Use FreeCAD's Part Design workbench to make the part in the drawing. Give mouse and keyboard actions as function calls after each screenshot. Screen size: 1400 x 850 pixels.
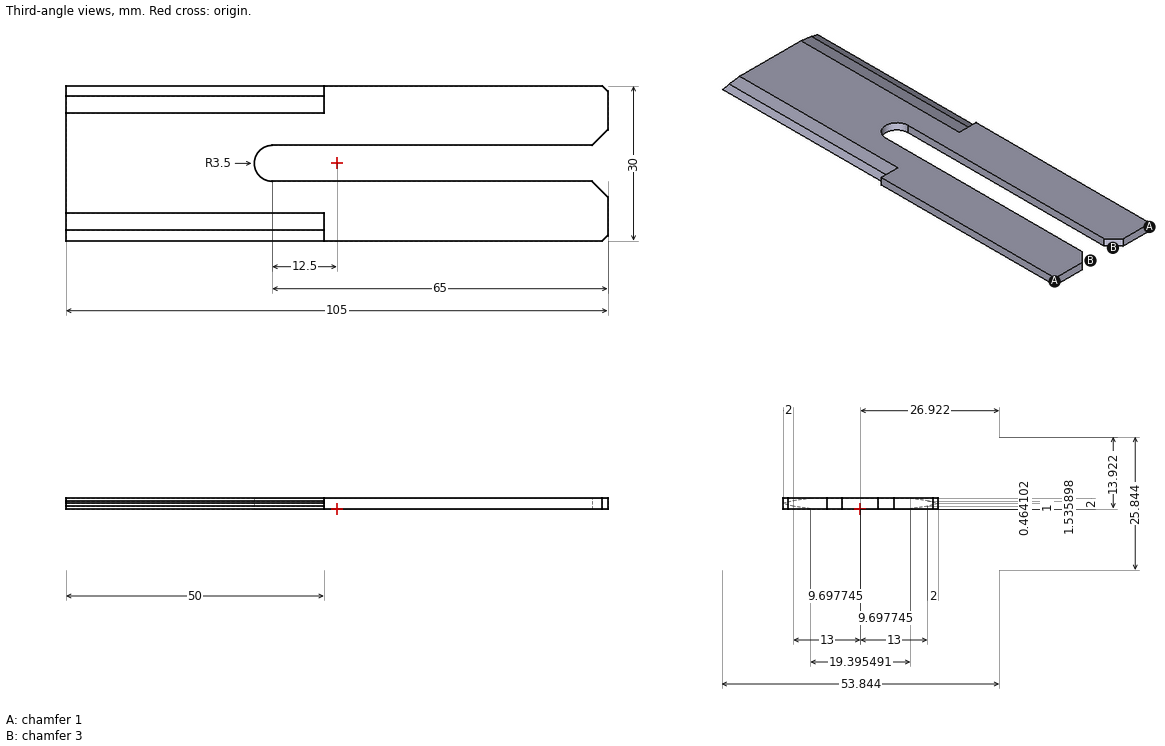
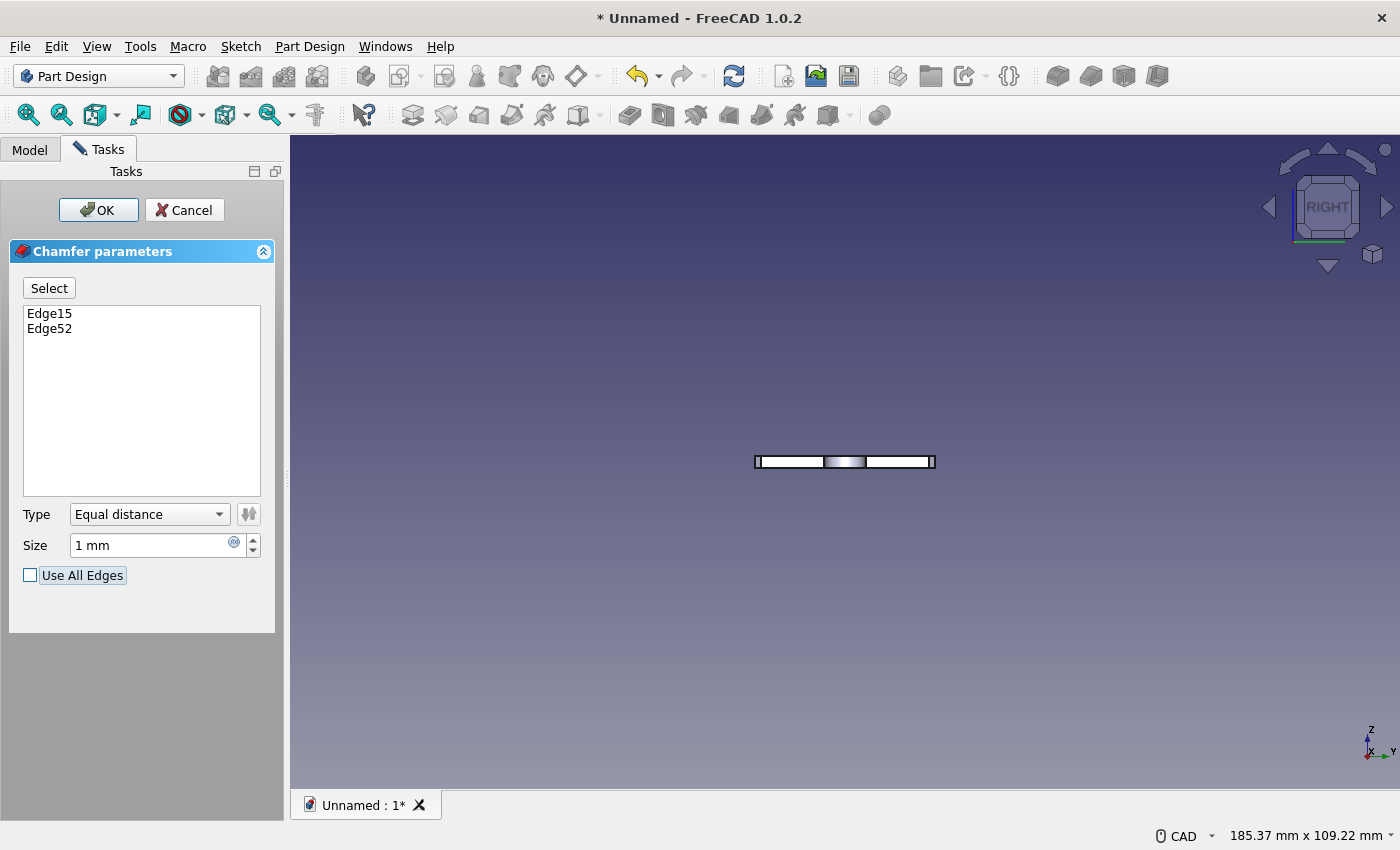
click(99, 210)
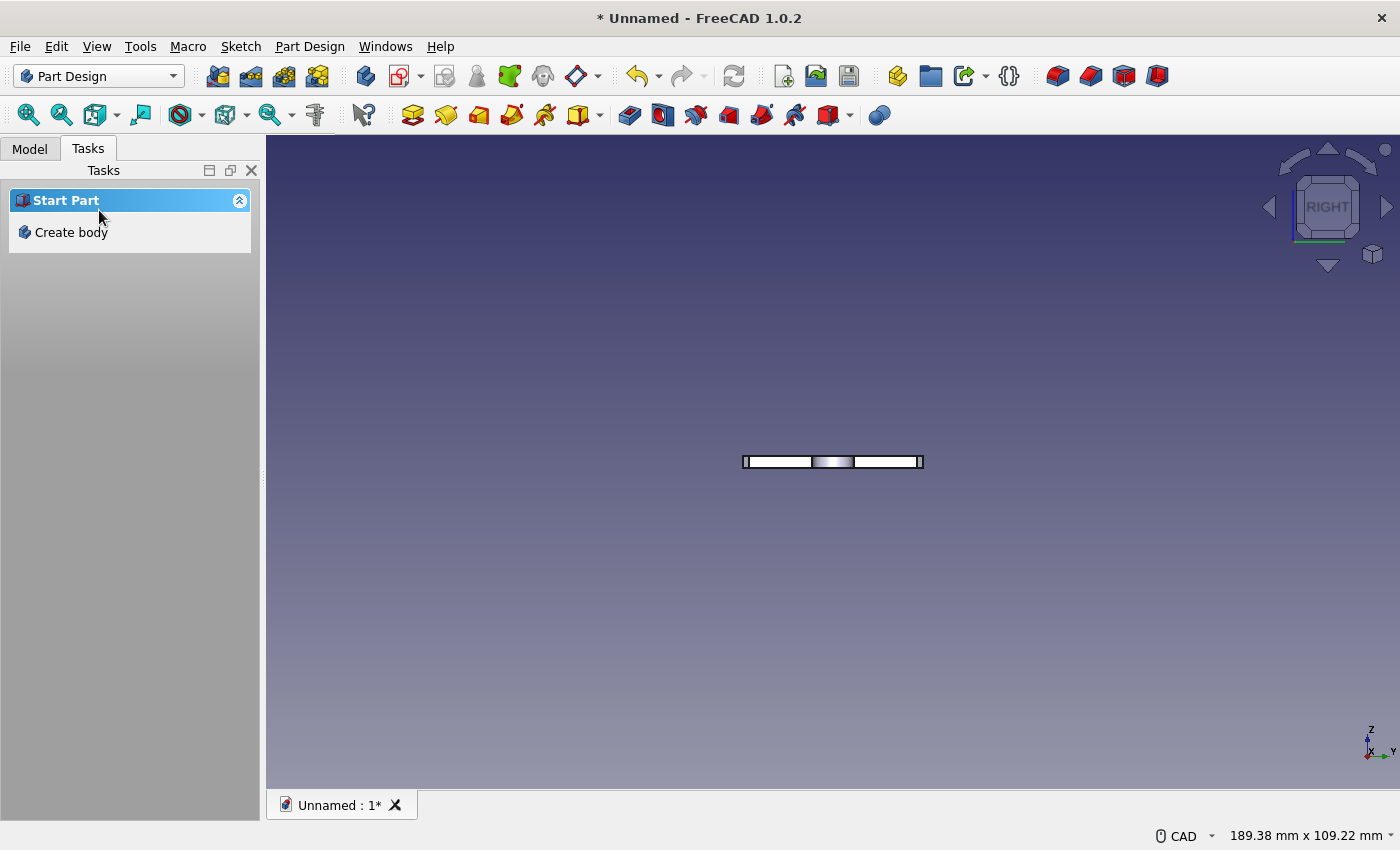
click(29, 116)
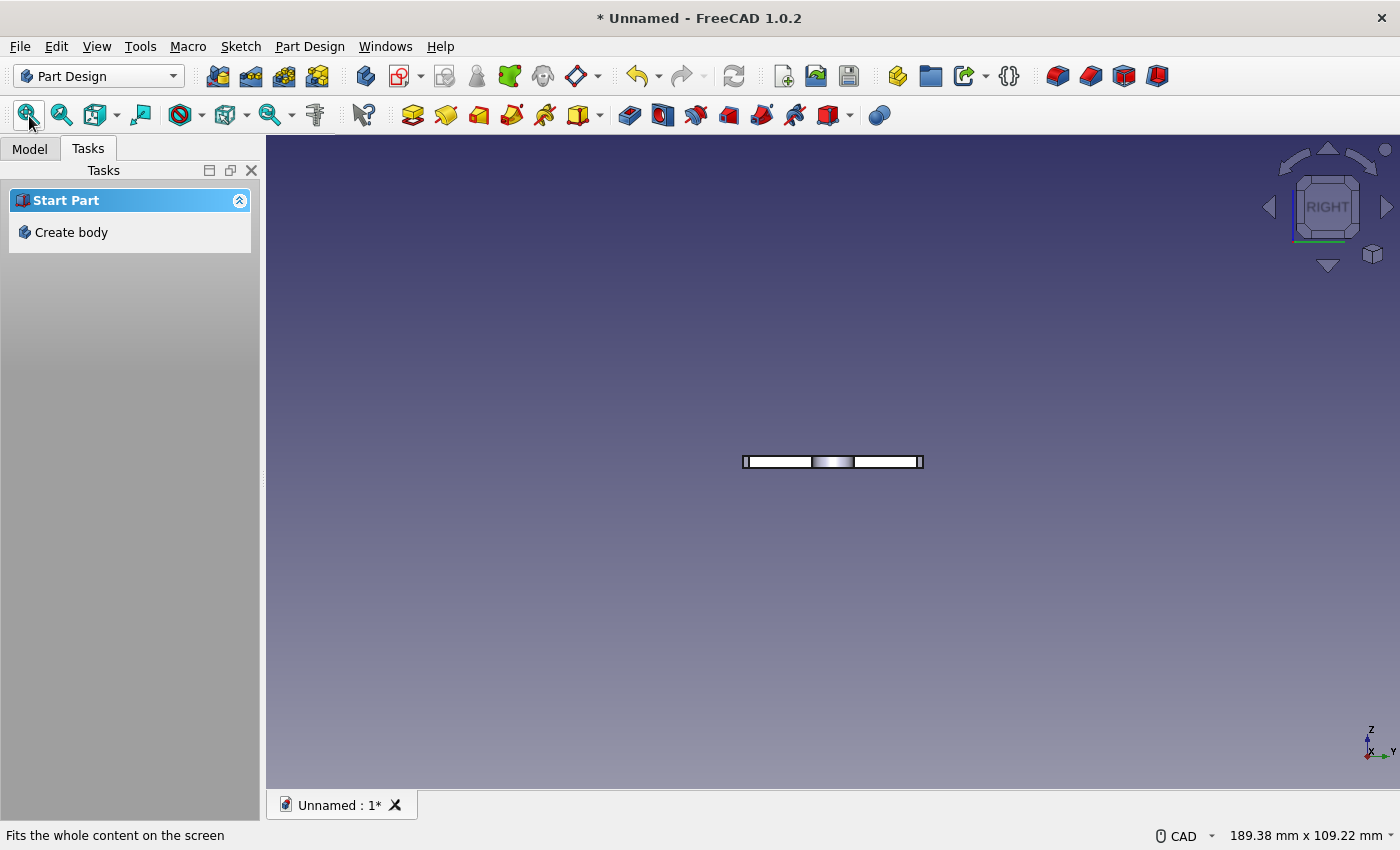
scroll(812, 461, up, 7)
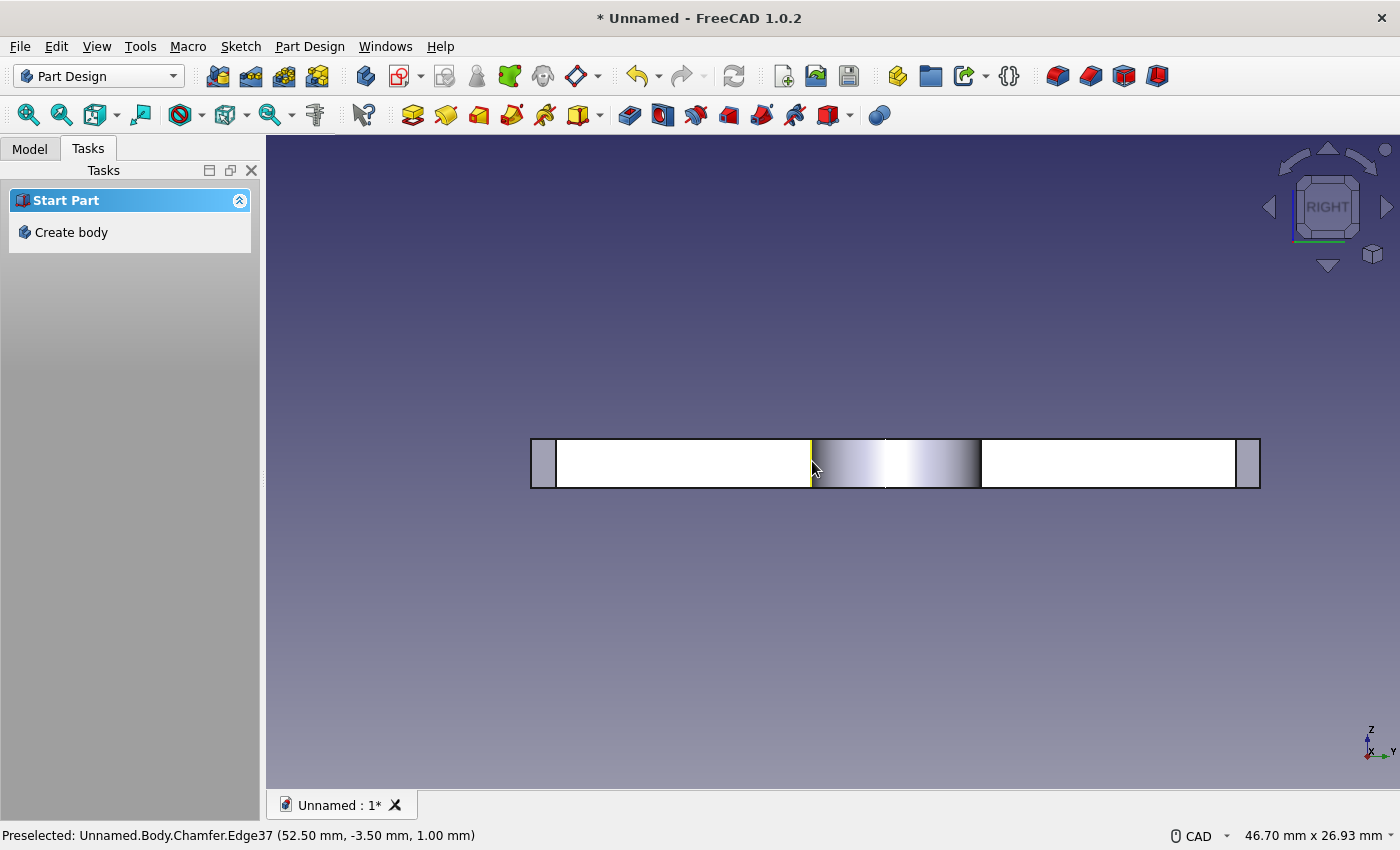
click(811, 463)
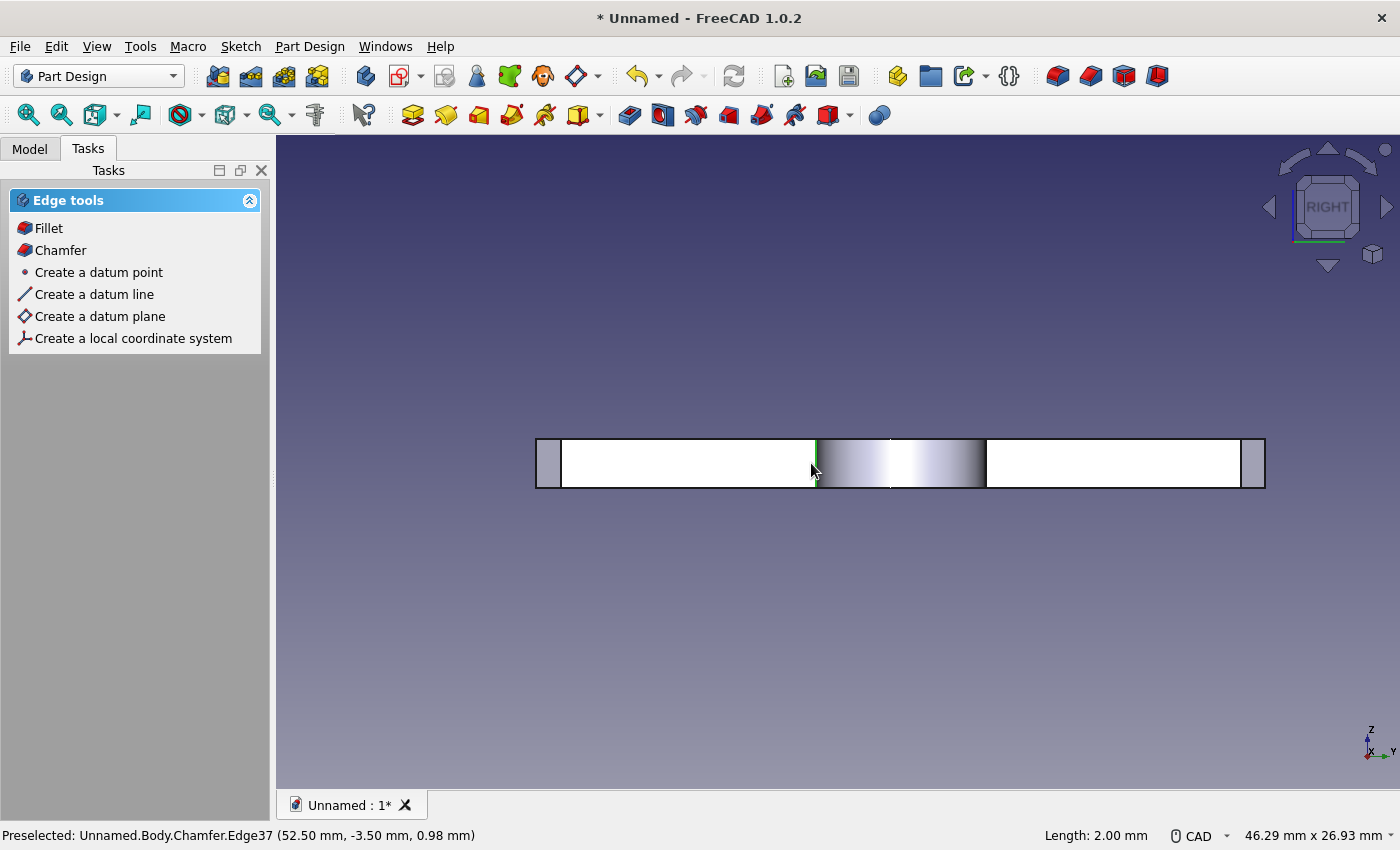
click(986, 463, ctrl)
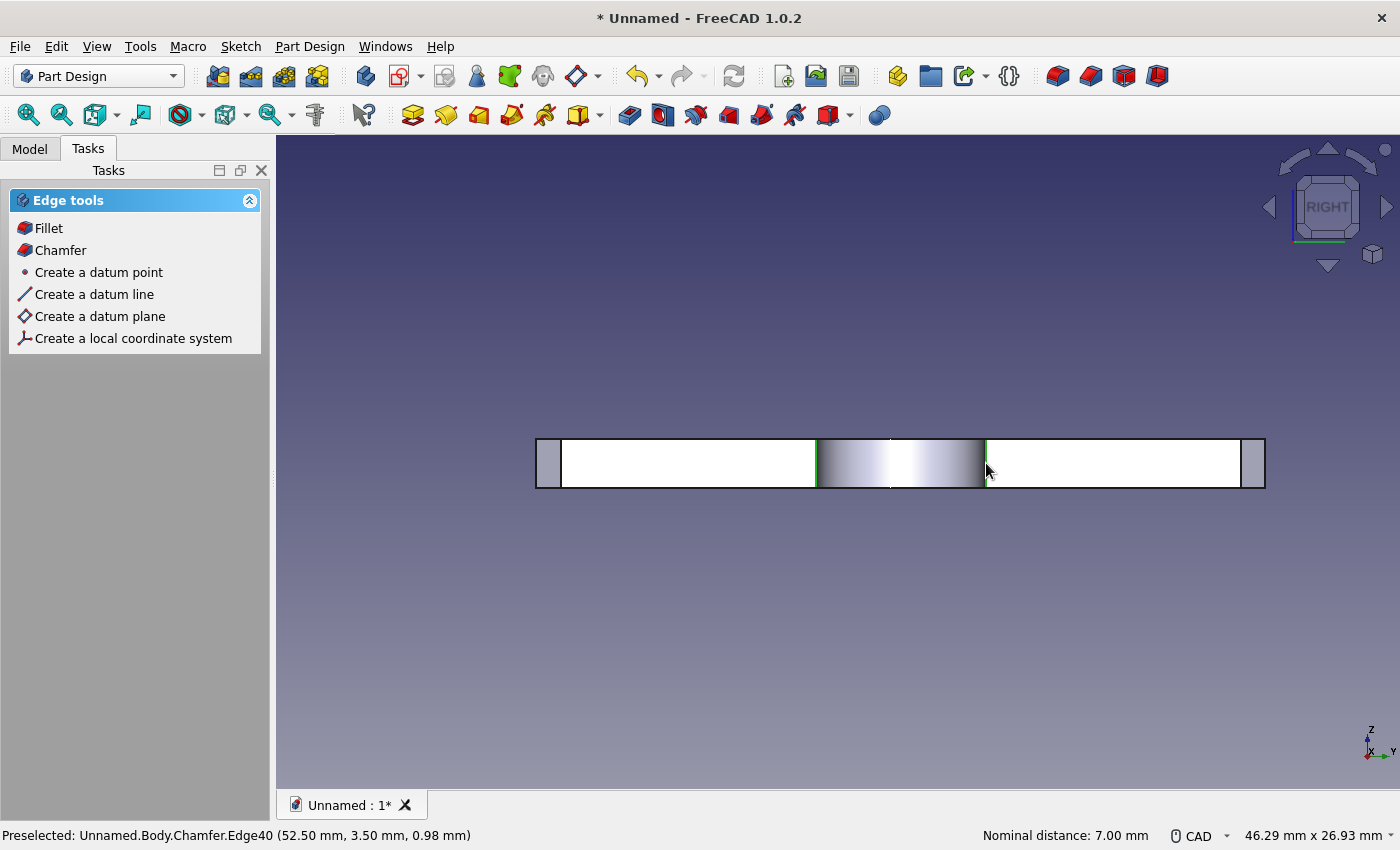
click(1091, 76)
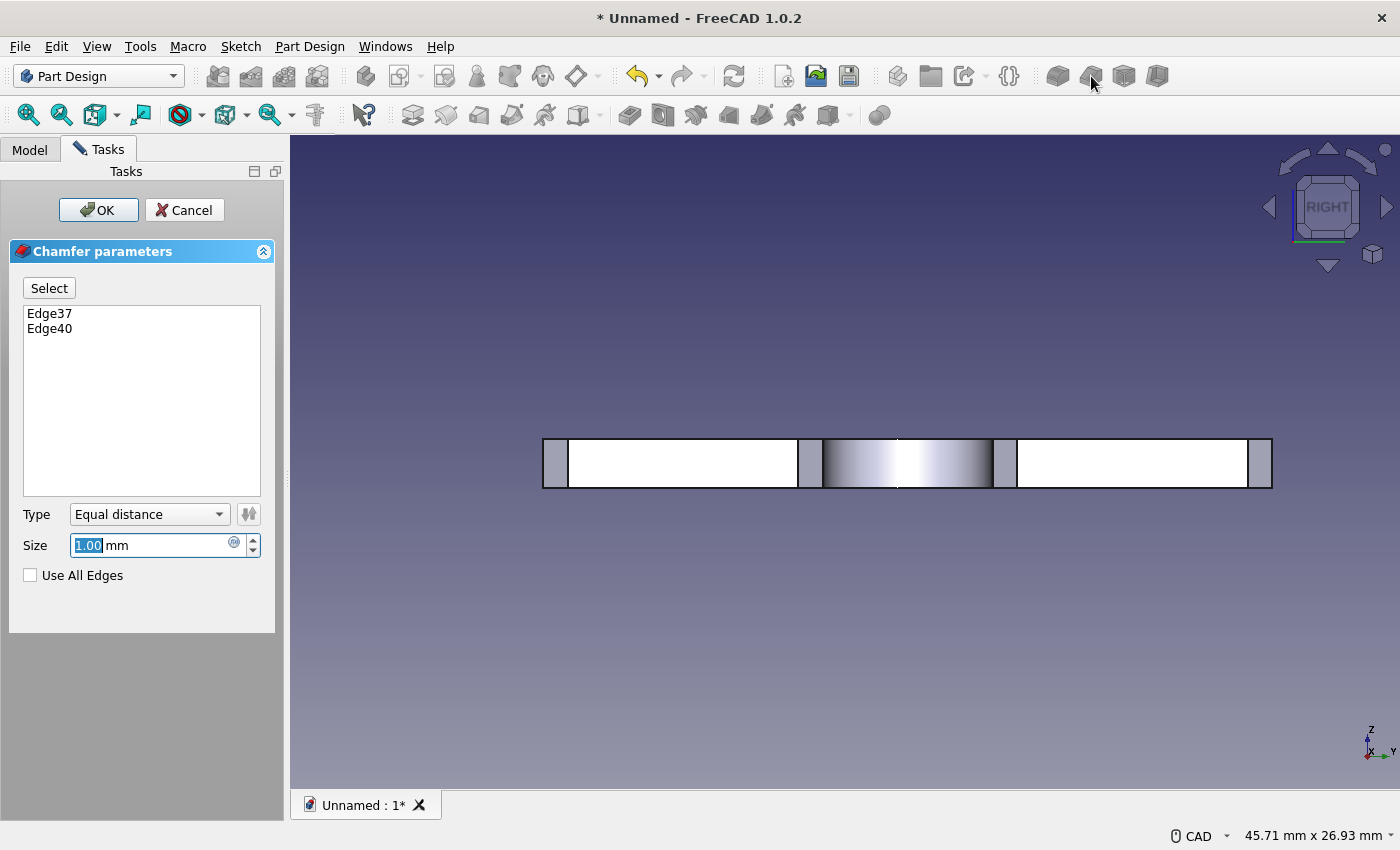
text(3)
key(Tab)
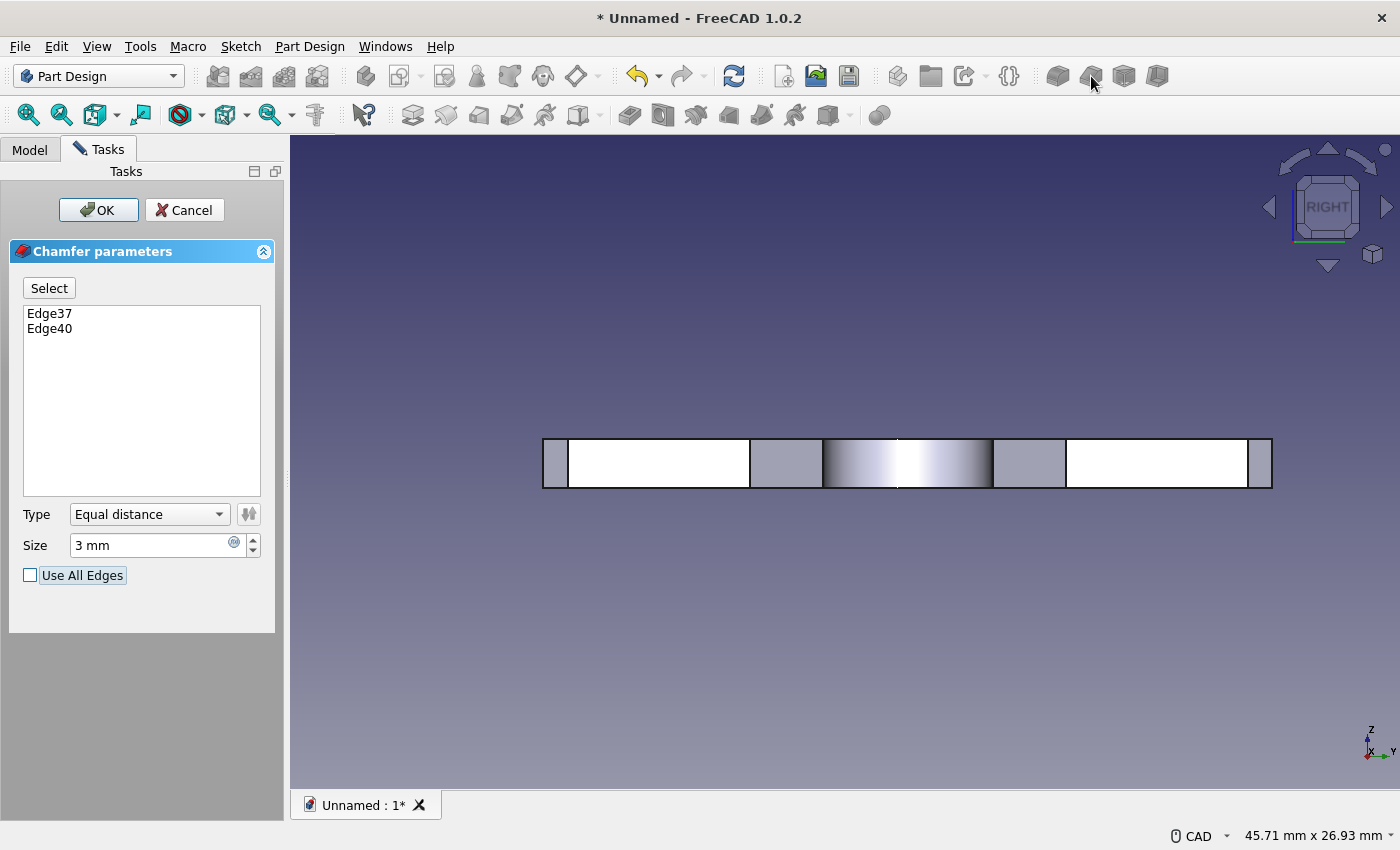
click(99, 210)